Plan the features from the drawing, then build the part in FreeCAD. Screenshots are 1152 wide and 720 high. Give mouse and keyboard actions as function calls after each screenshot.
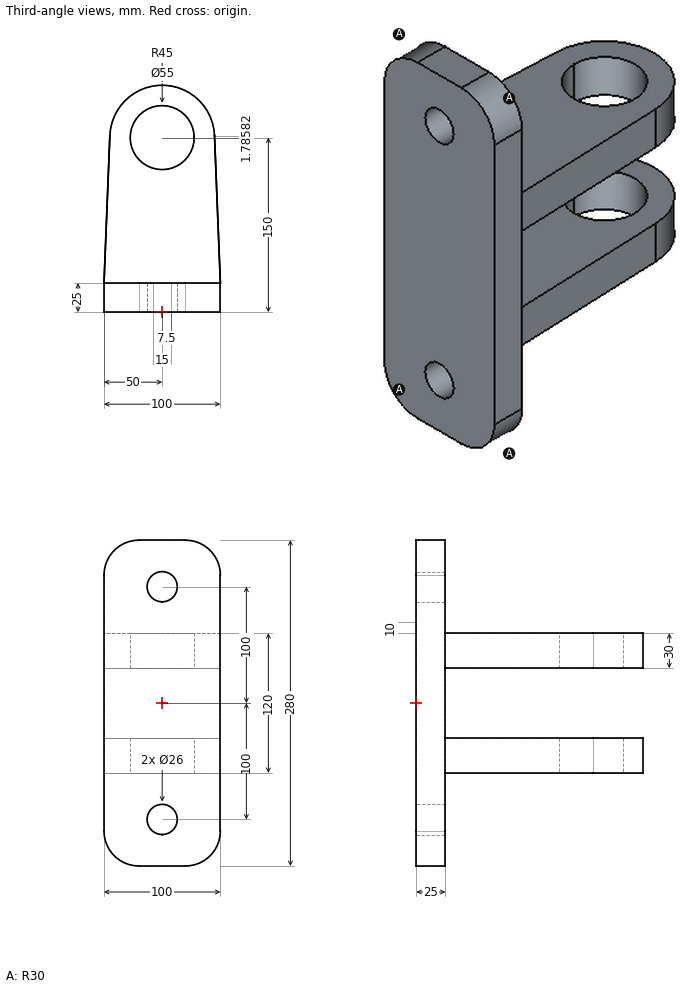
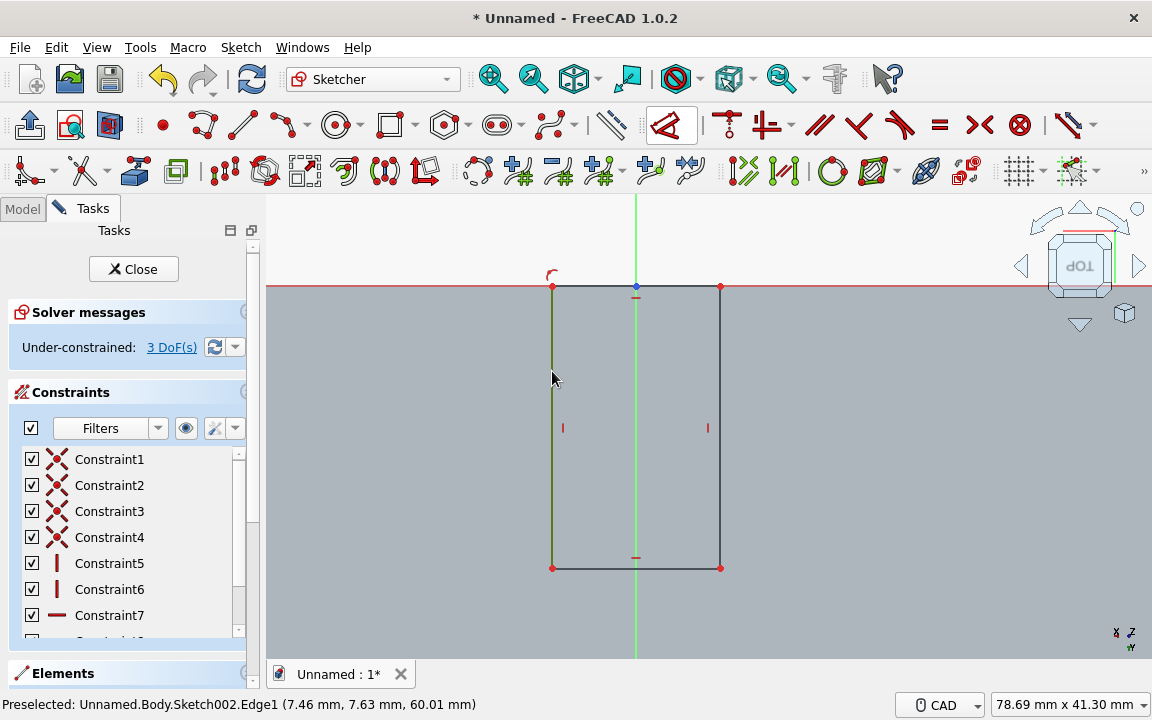
key(i)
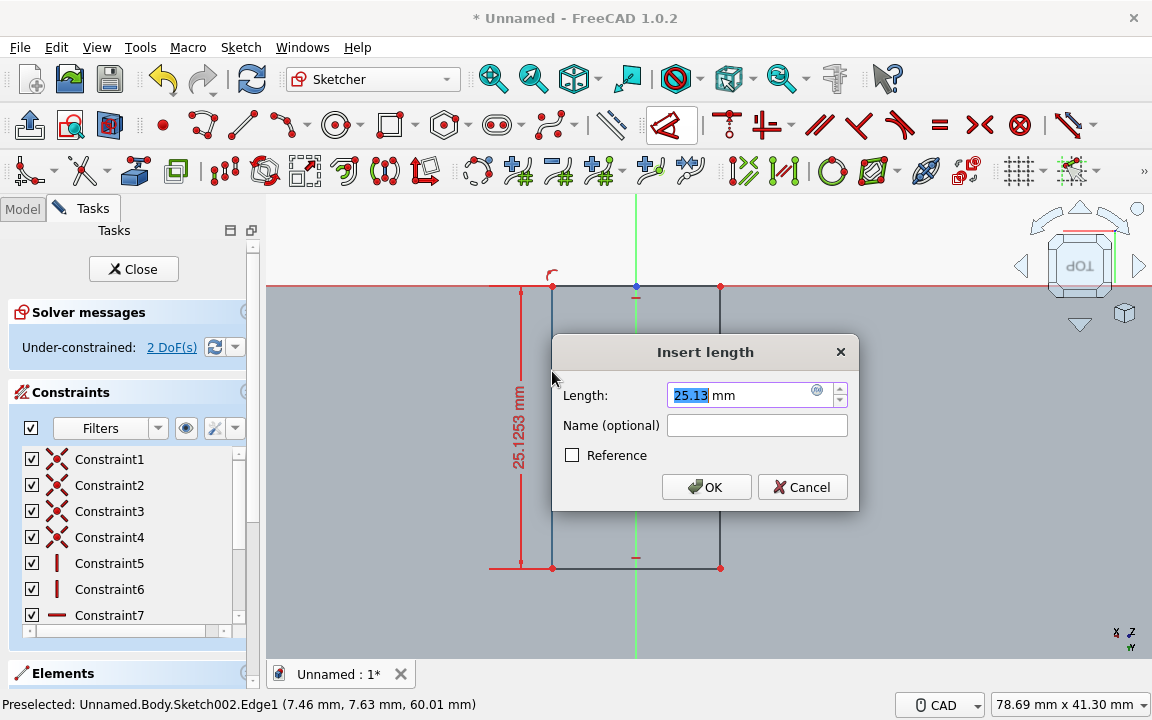
text(25)
key(Return)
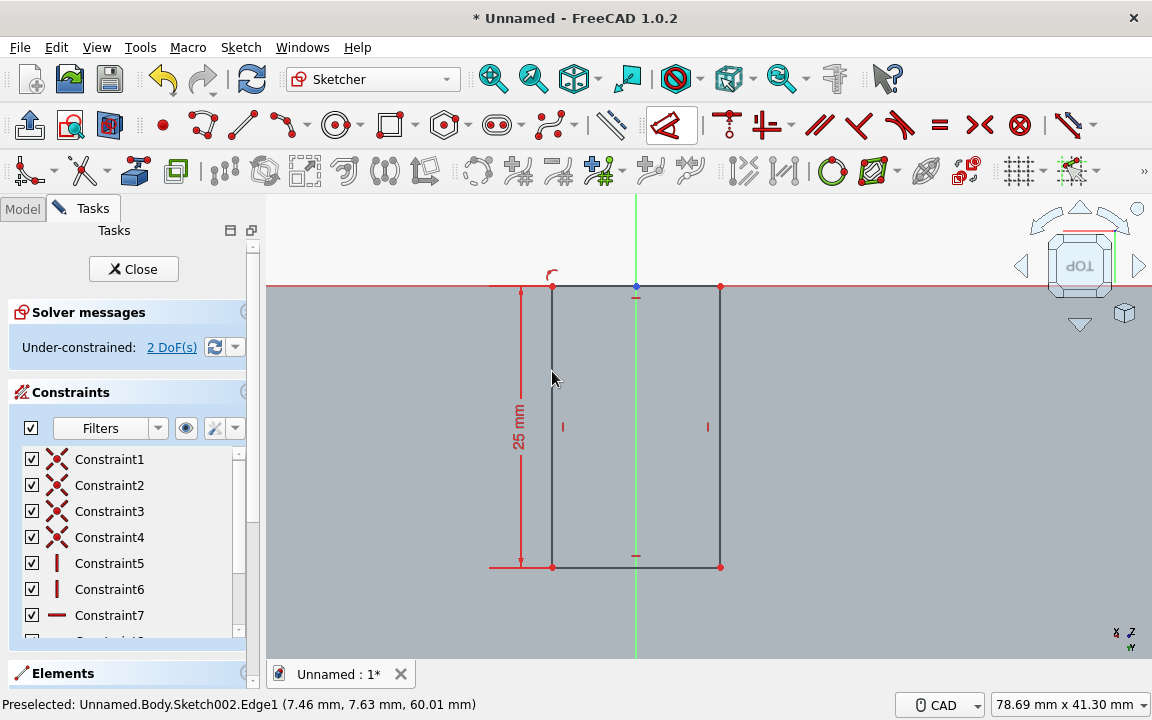
click(602, 568)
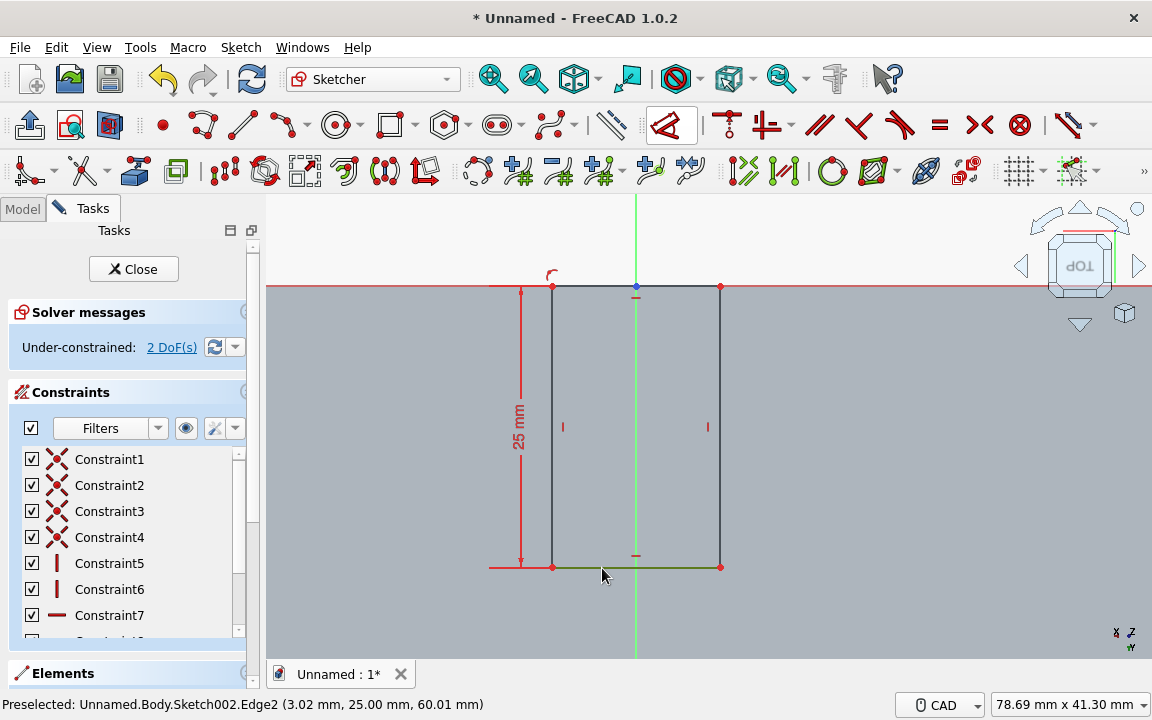
click(692, 126)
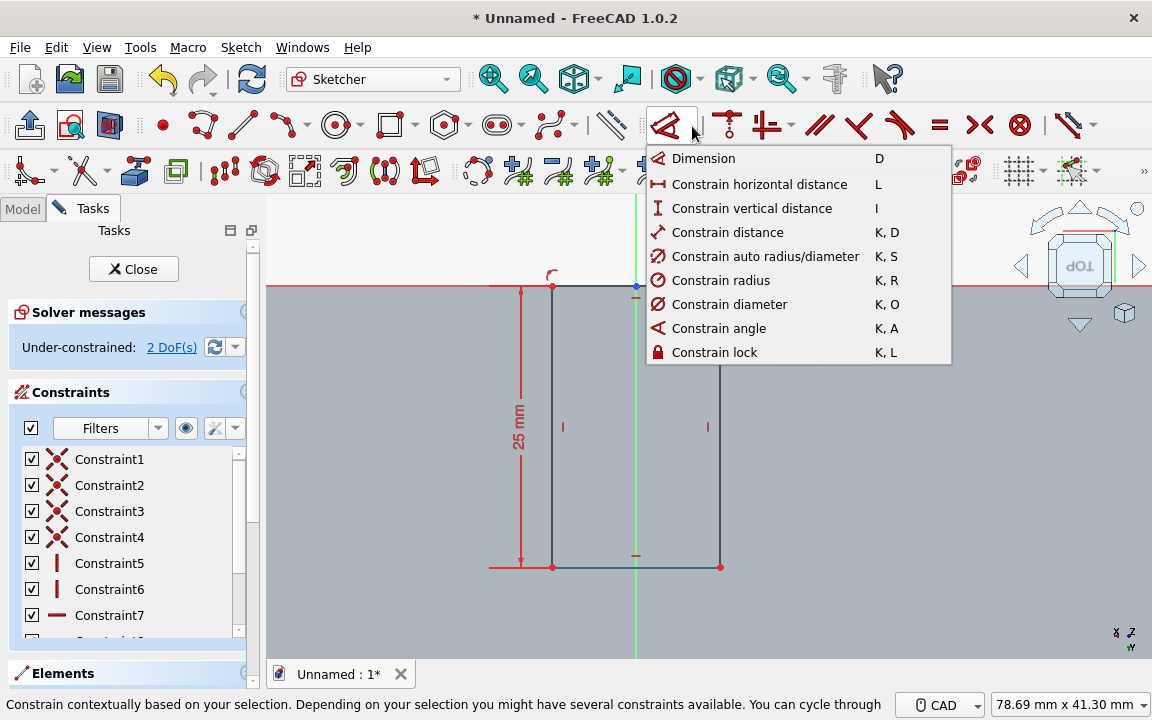
click(799, 184)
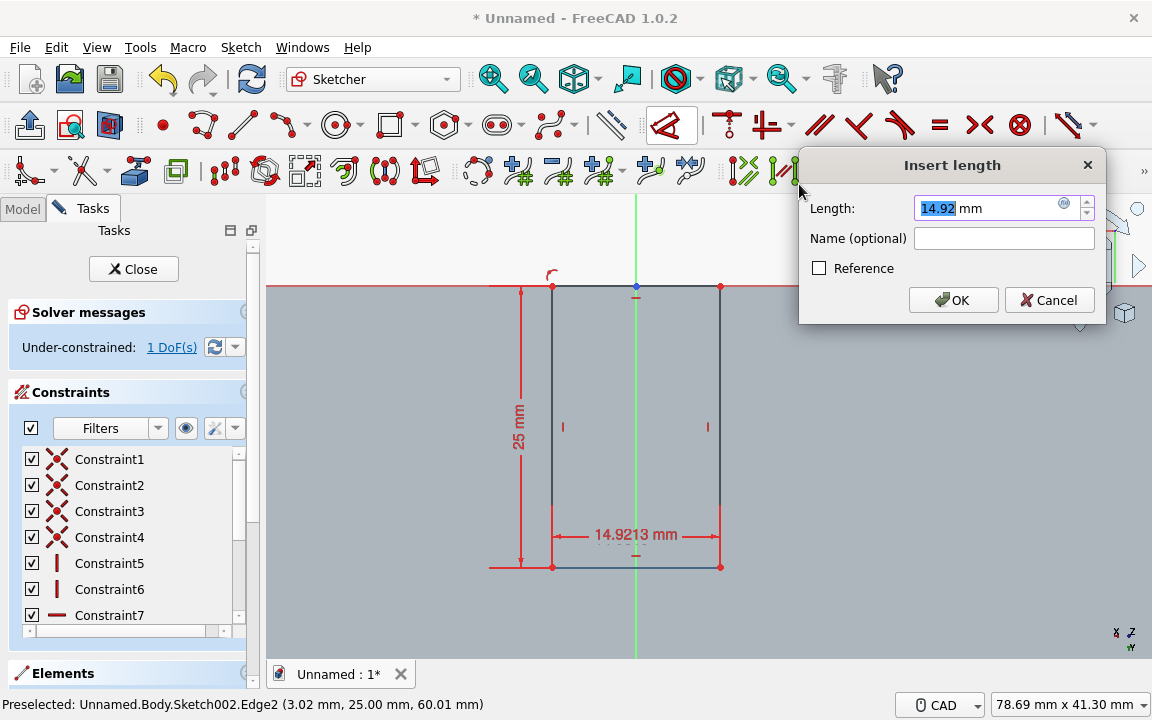
text(15)
key(Return)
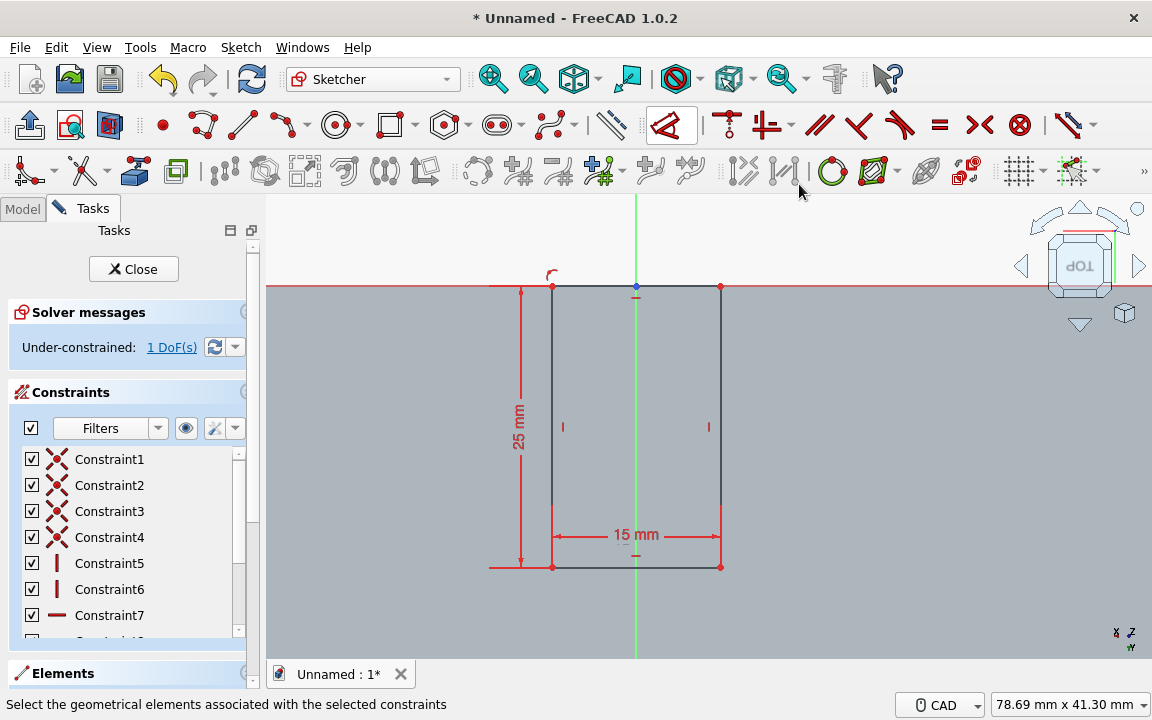
click(552, 286)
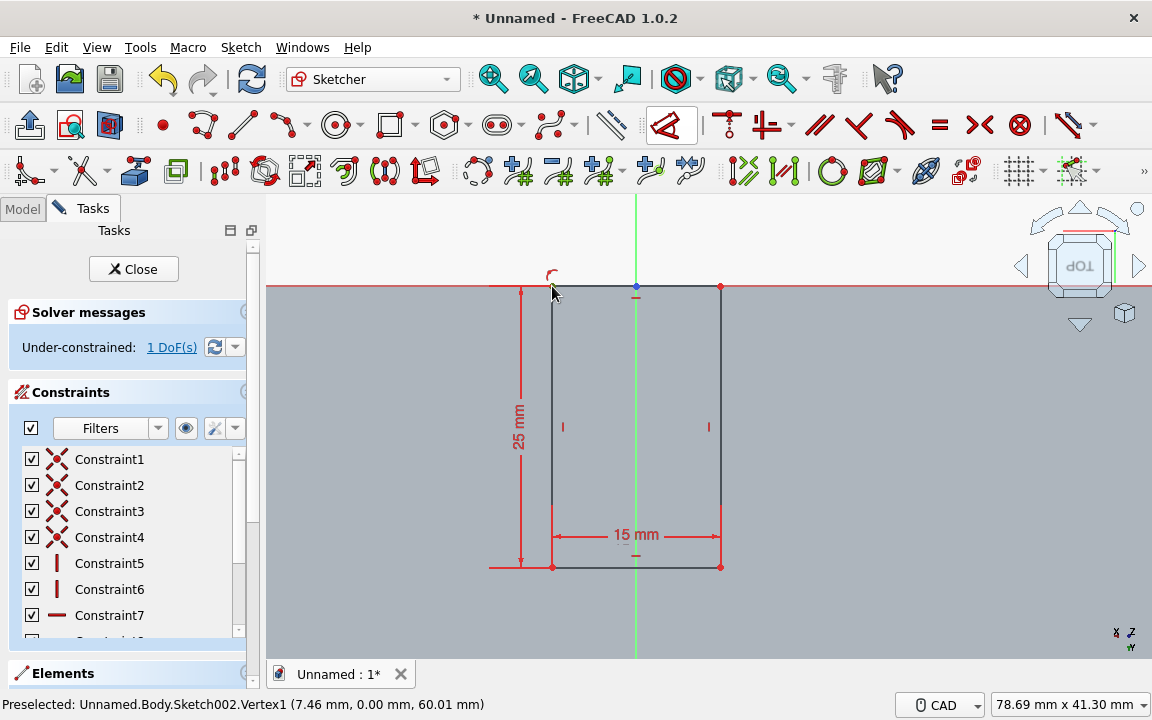
click(692, 126)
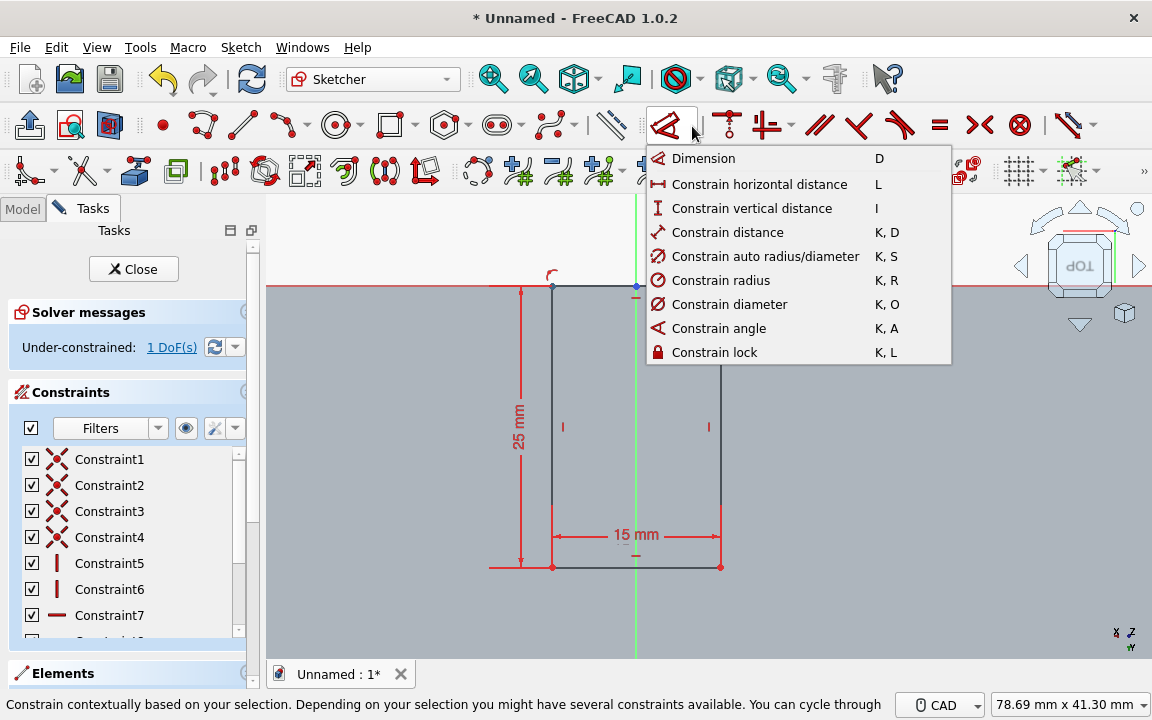
click(799, 184)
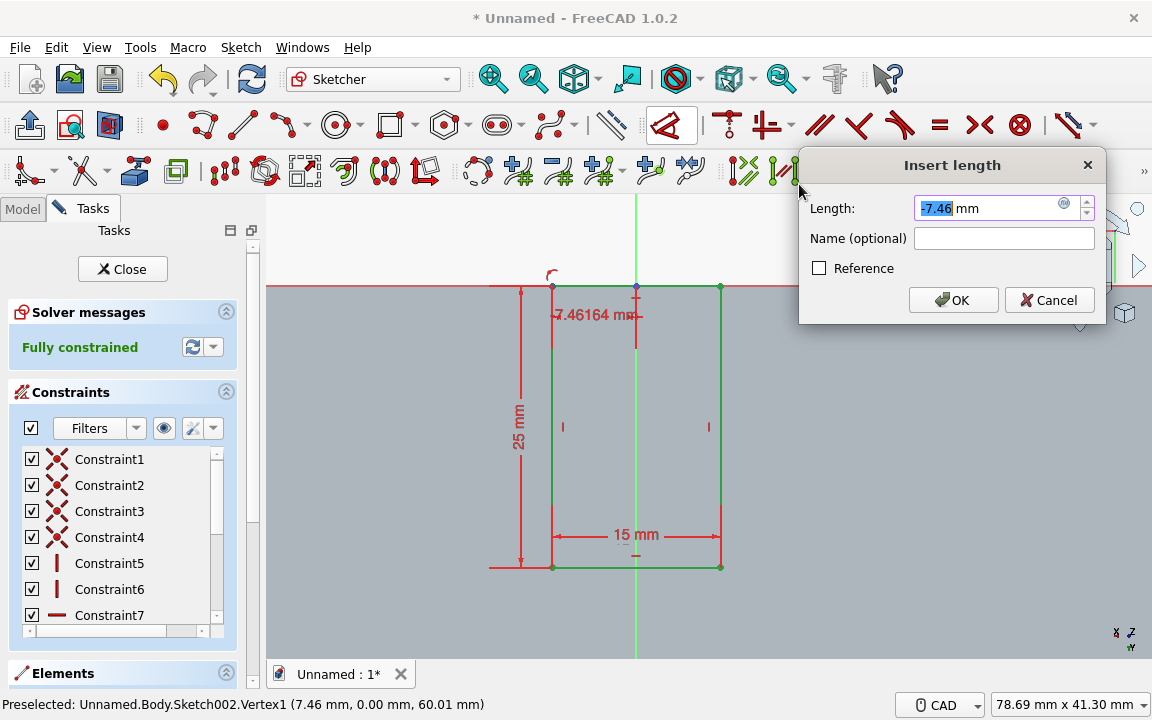
text(-7.5)
key(Return)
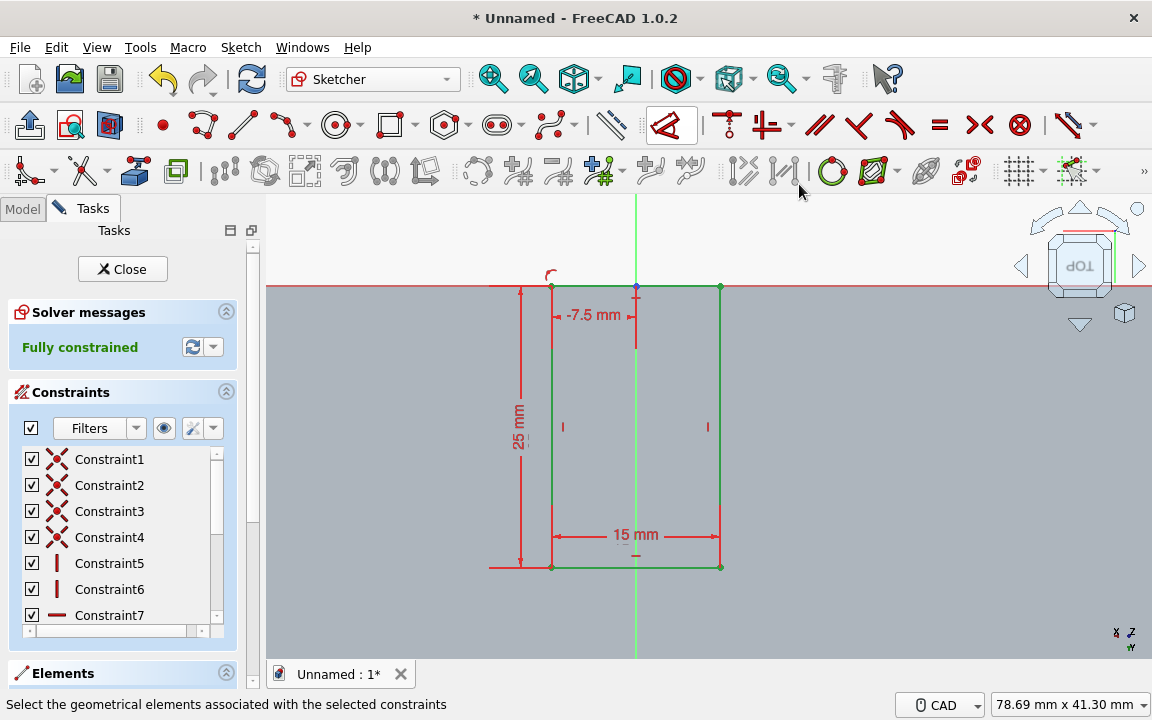
click(123, 269)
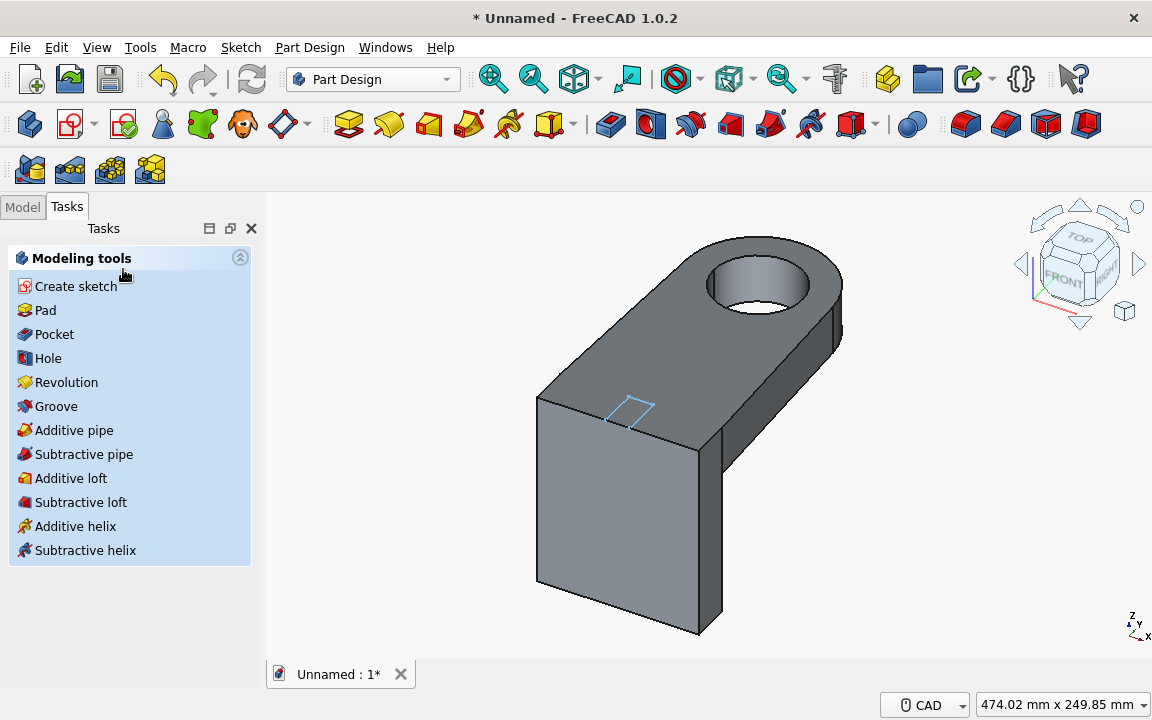
click(350, 124)